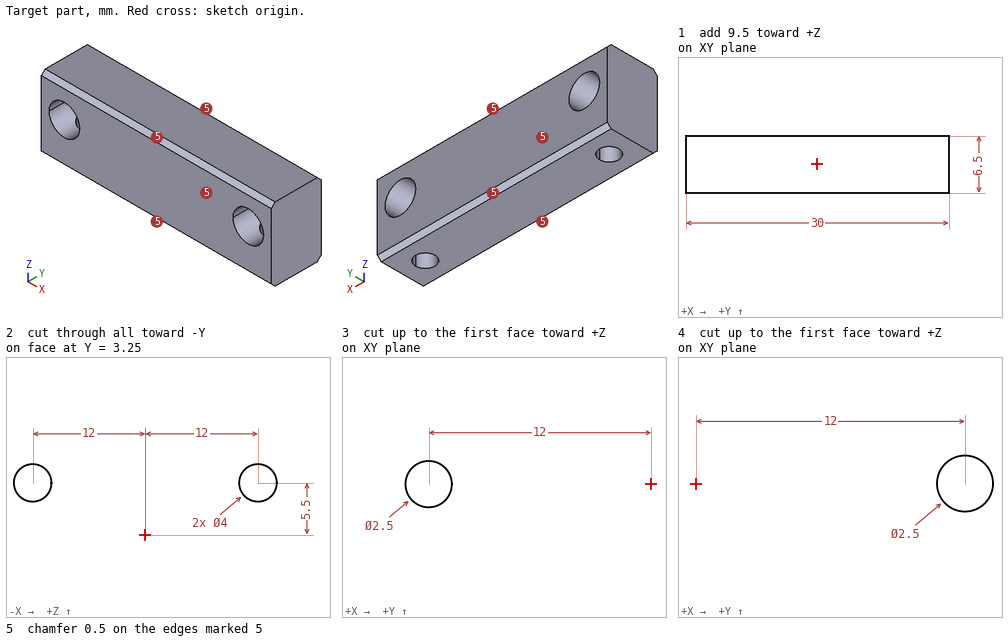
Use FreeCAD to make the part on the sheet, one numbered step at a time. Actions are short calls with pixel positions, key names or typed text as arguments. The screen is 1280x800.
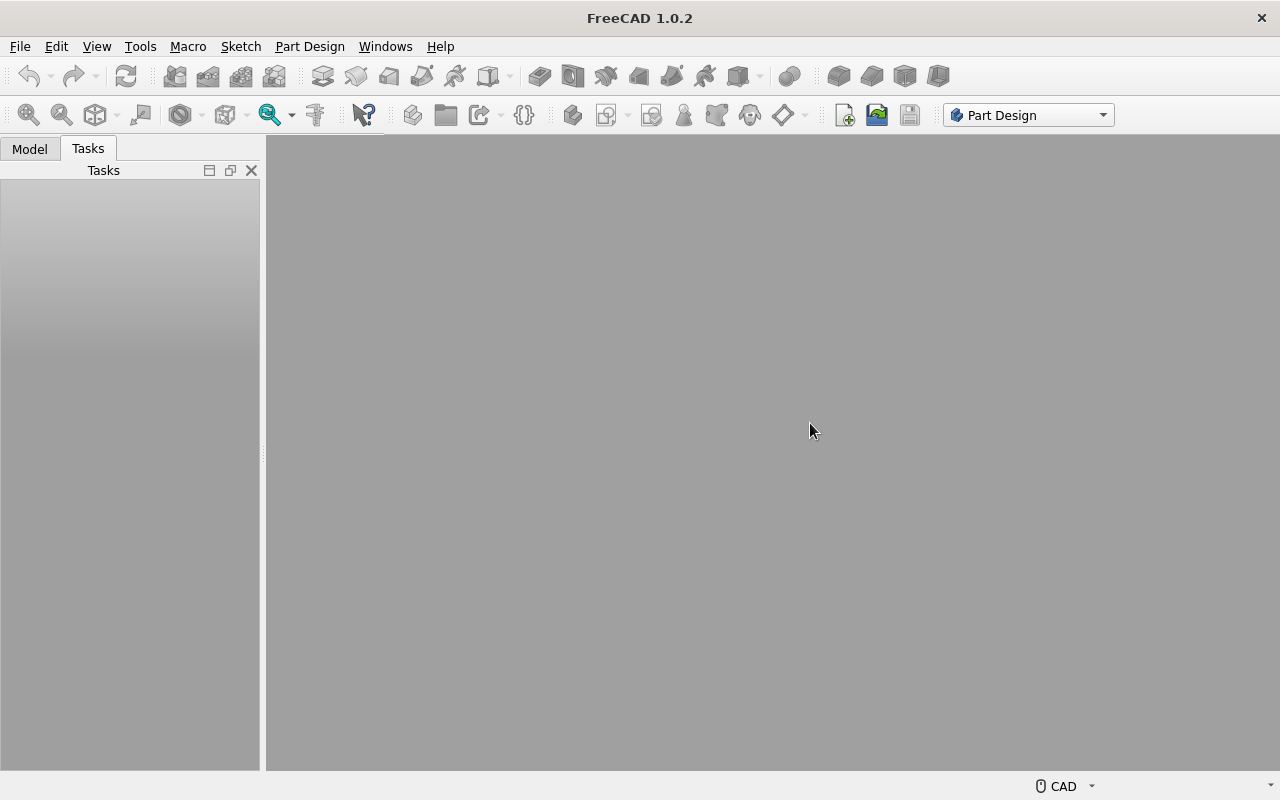
click(844, 116)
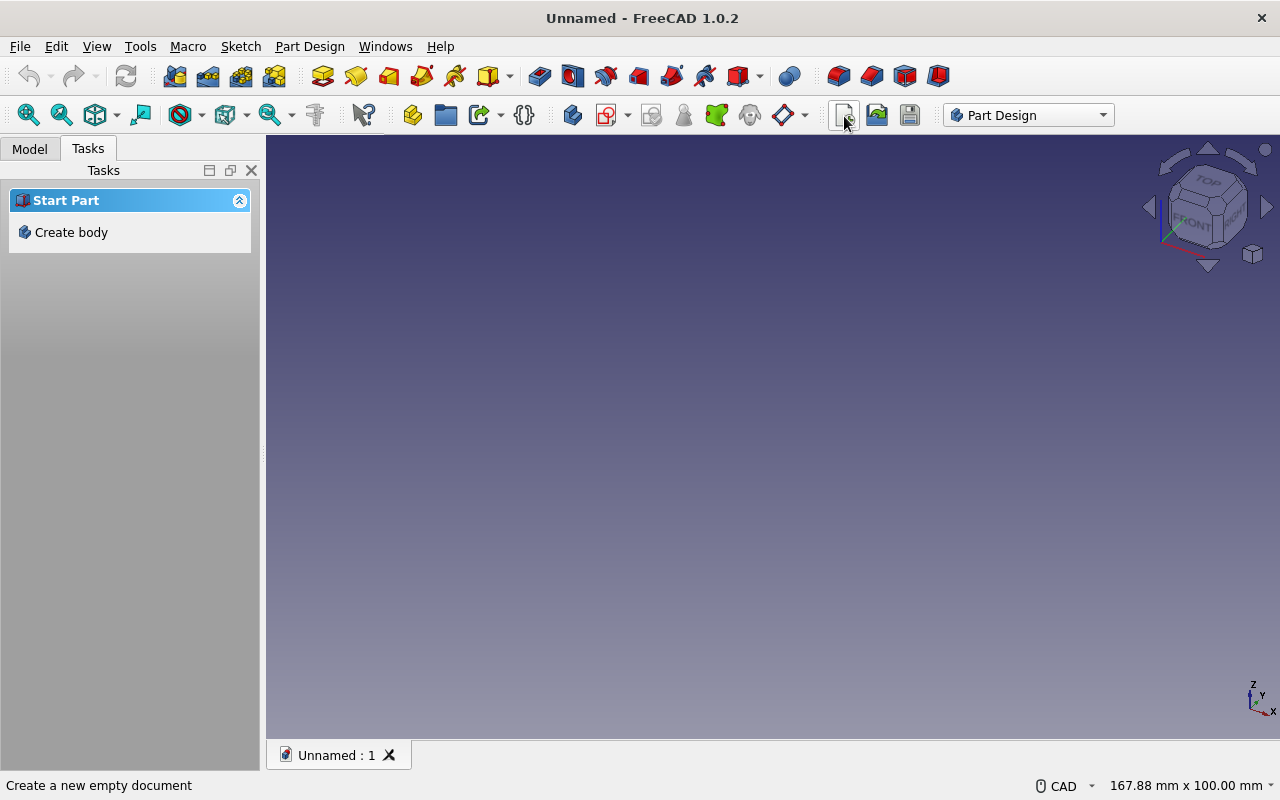
click(606, 116)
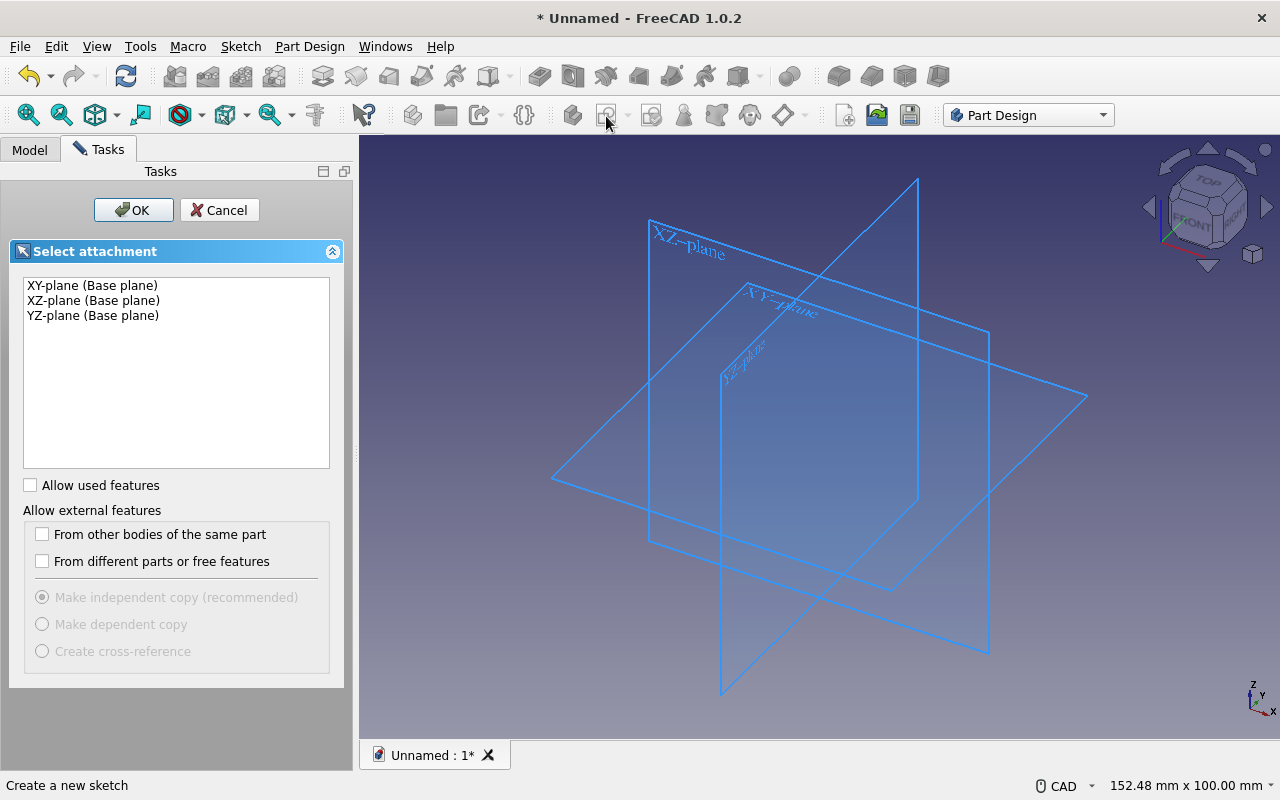
click(84, 286)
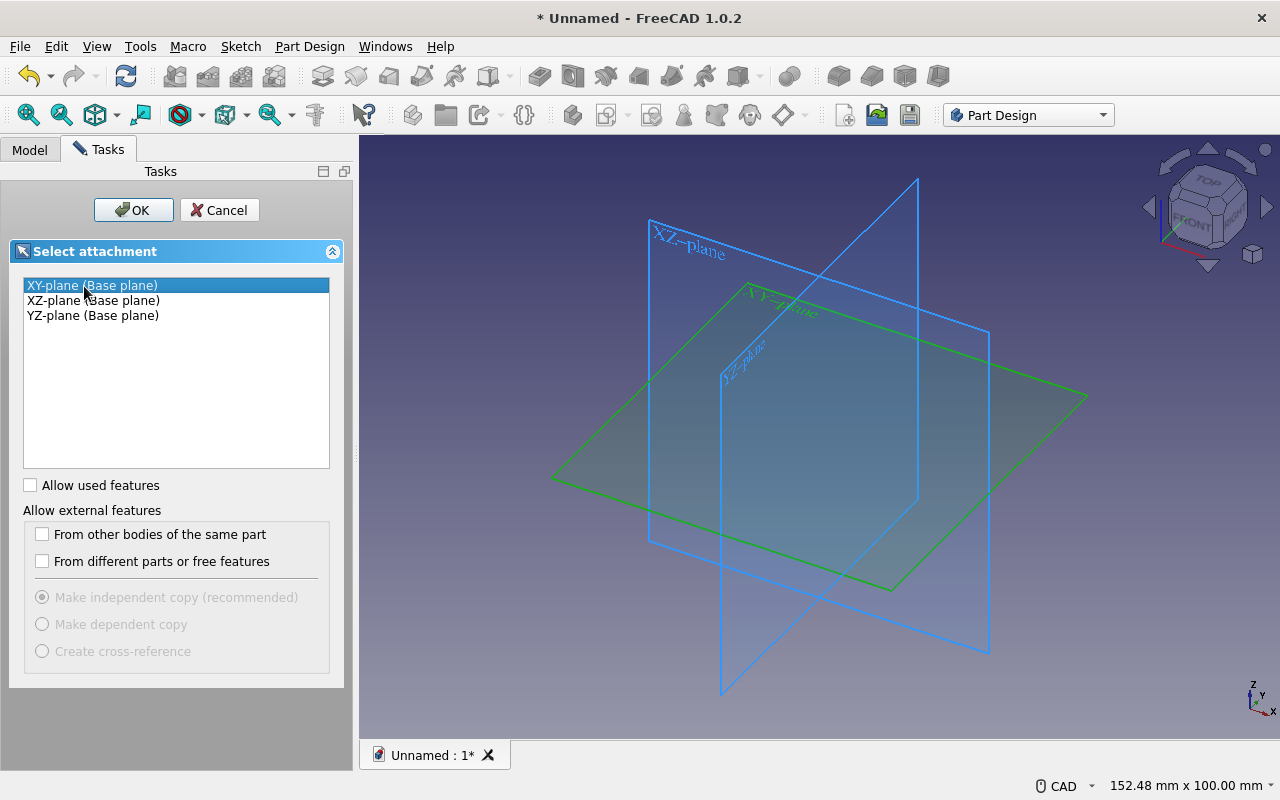
click(134, 210)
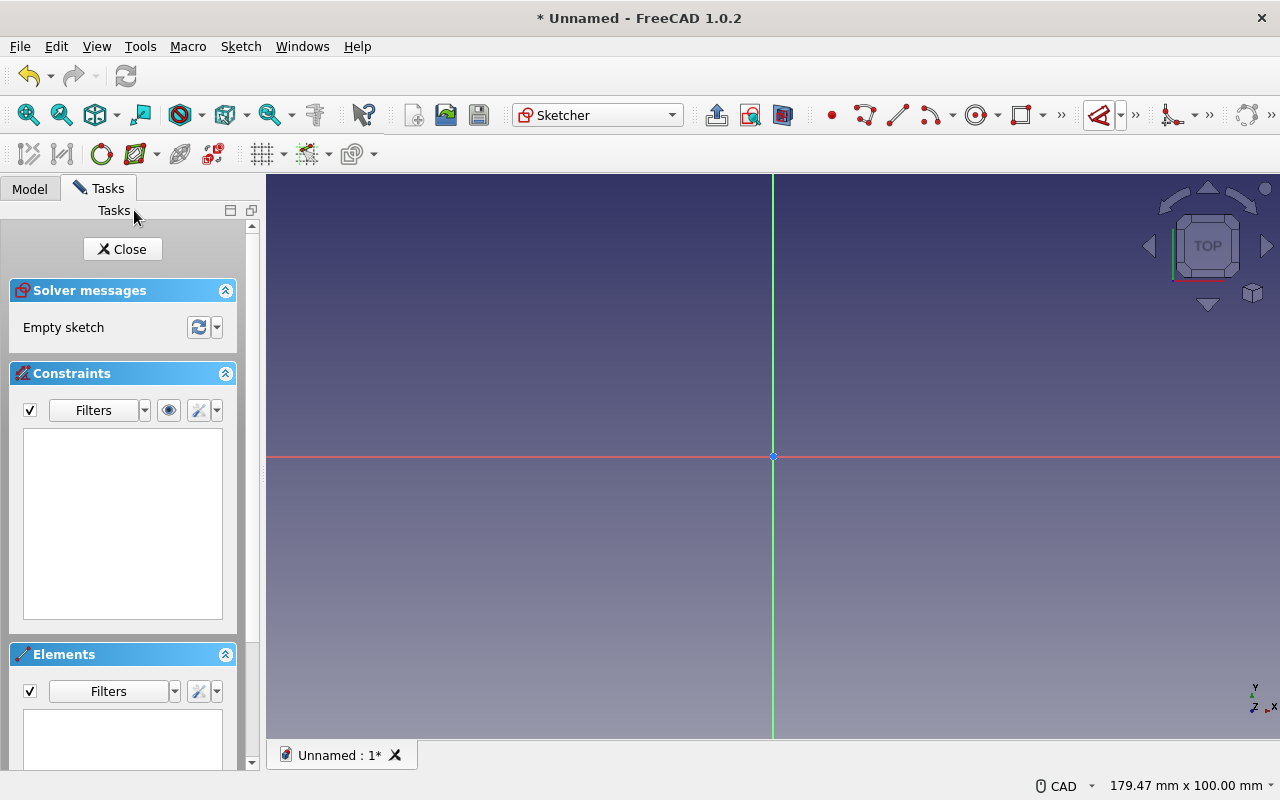
scroll(803, 456, up, 6)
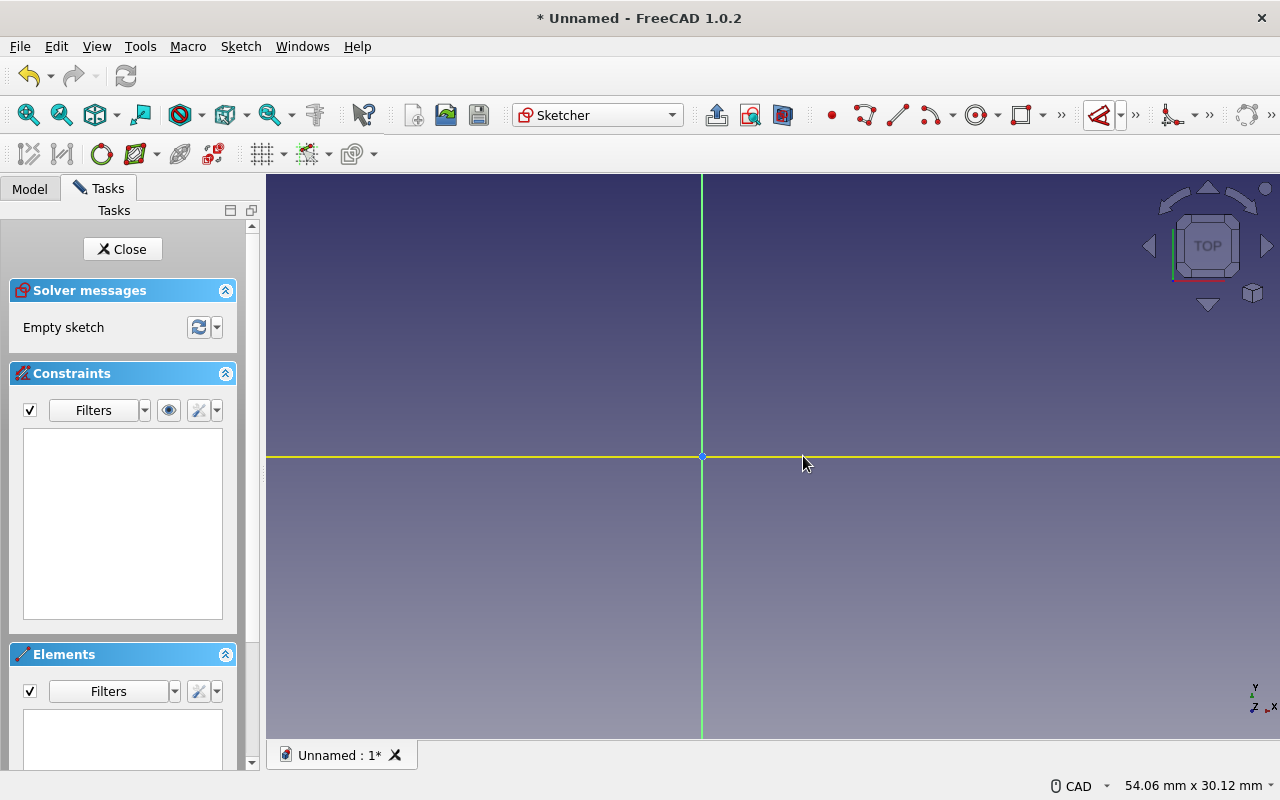
key(g)
key(v)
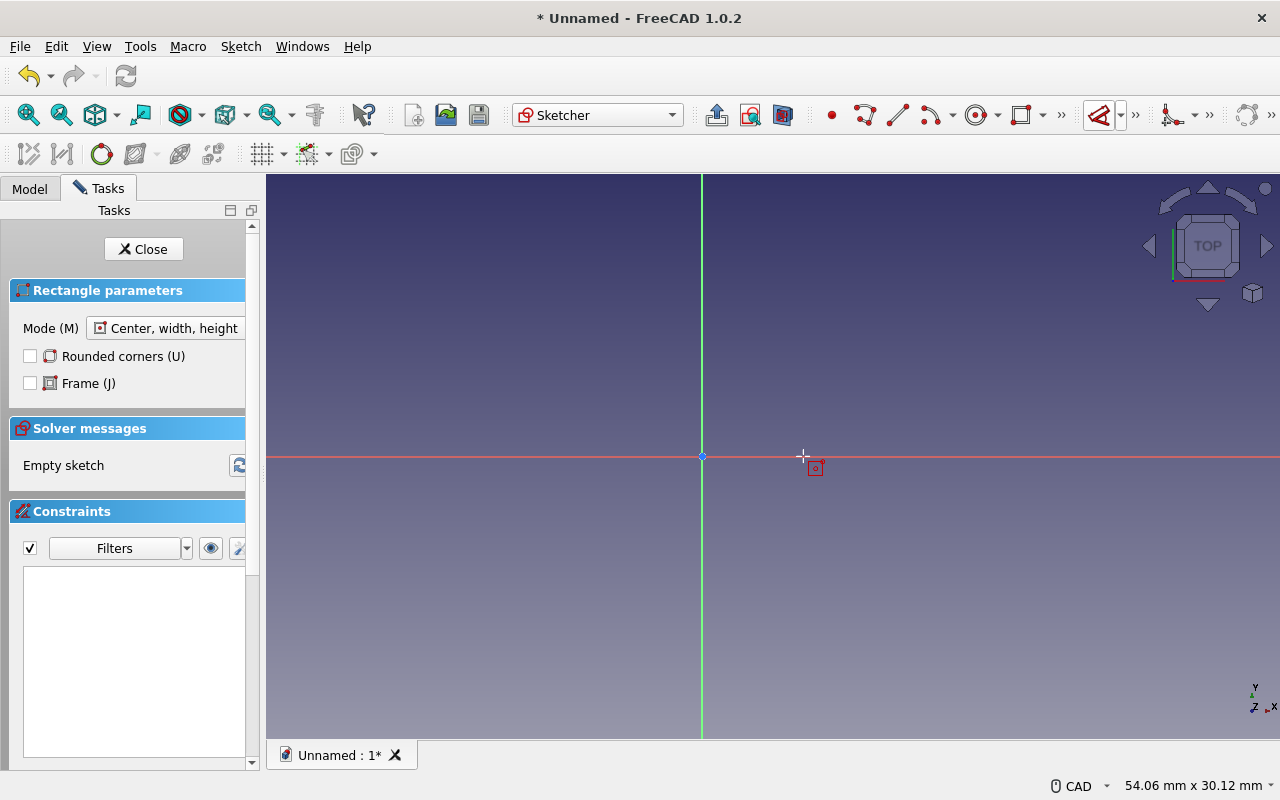
click(702, 456)
click(984, 396)
key(Escape)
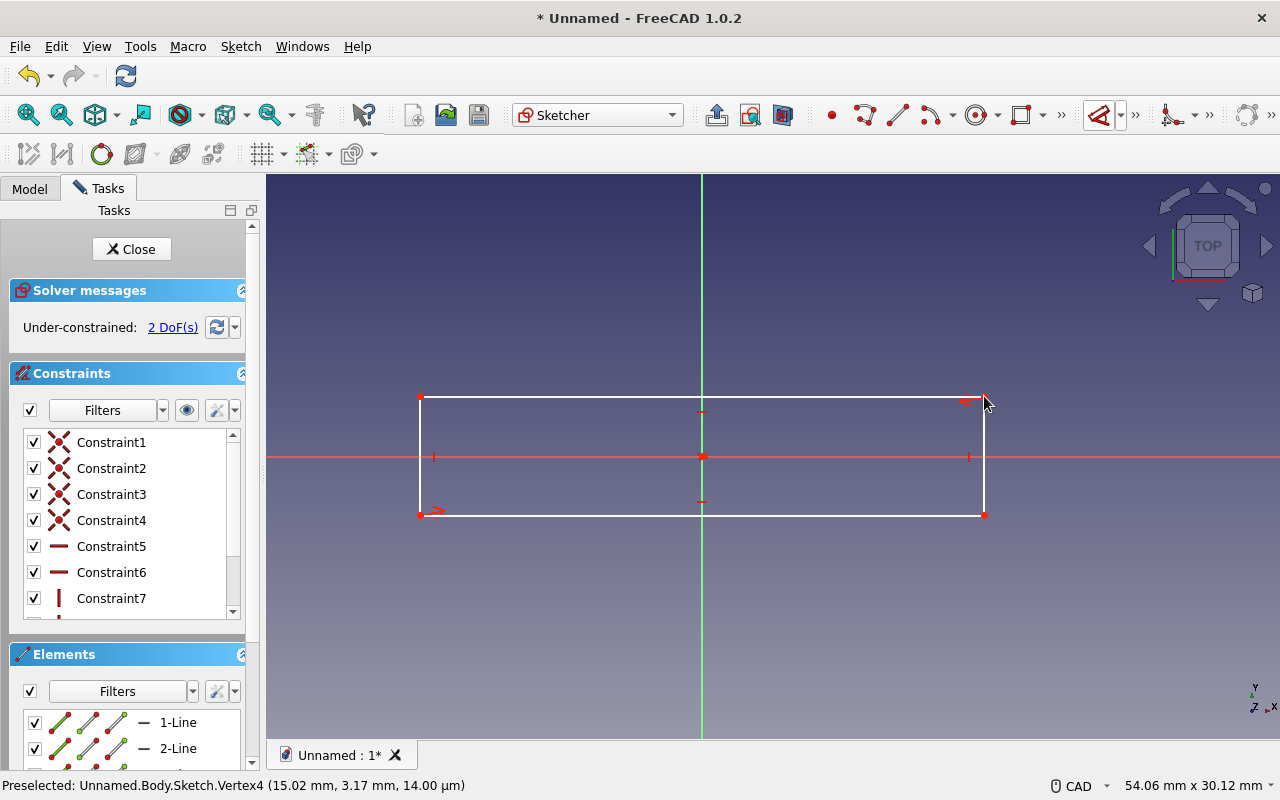
click(1098, 116)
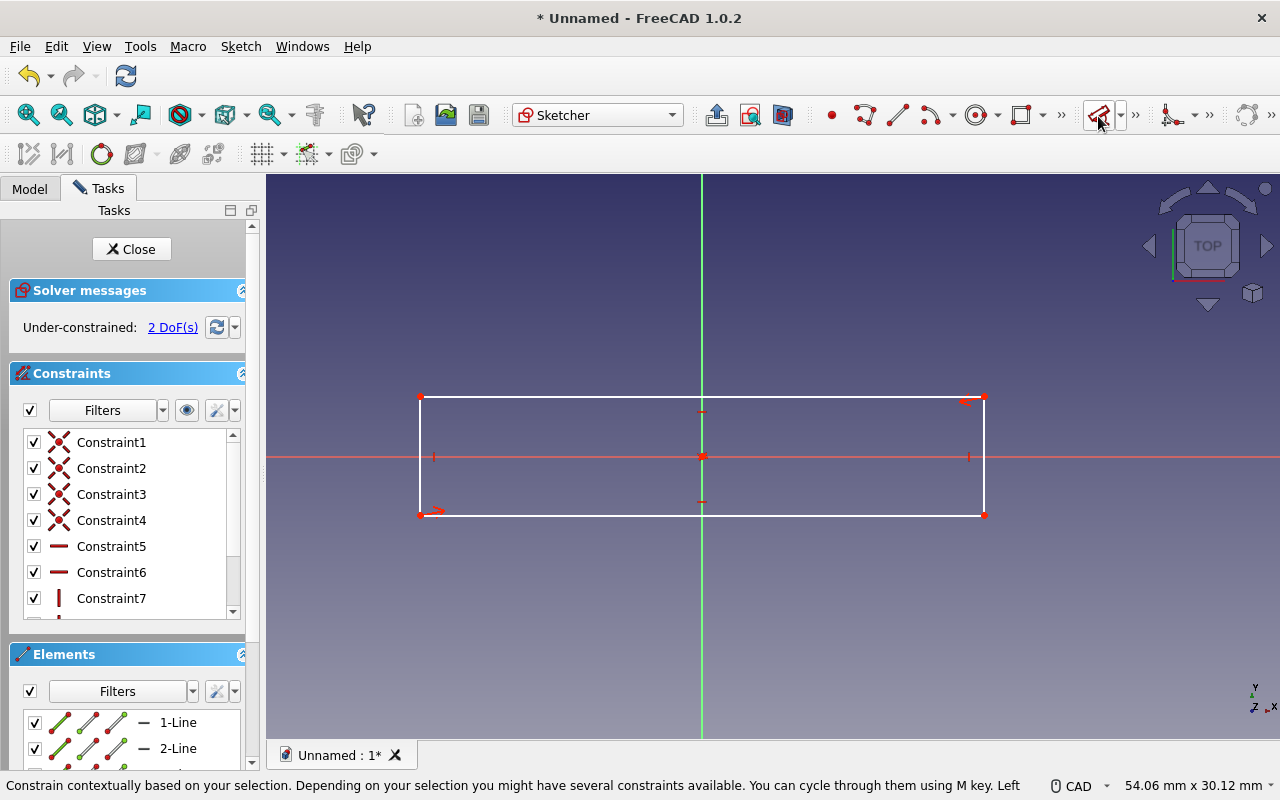
click(589, 516)
click(573, 550)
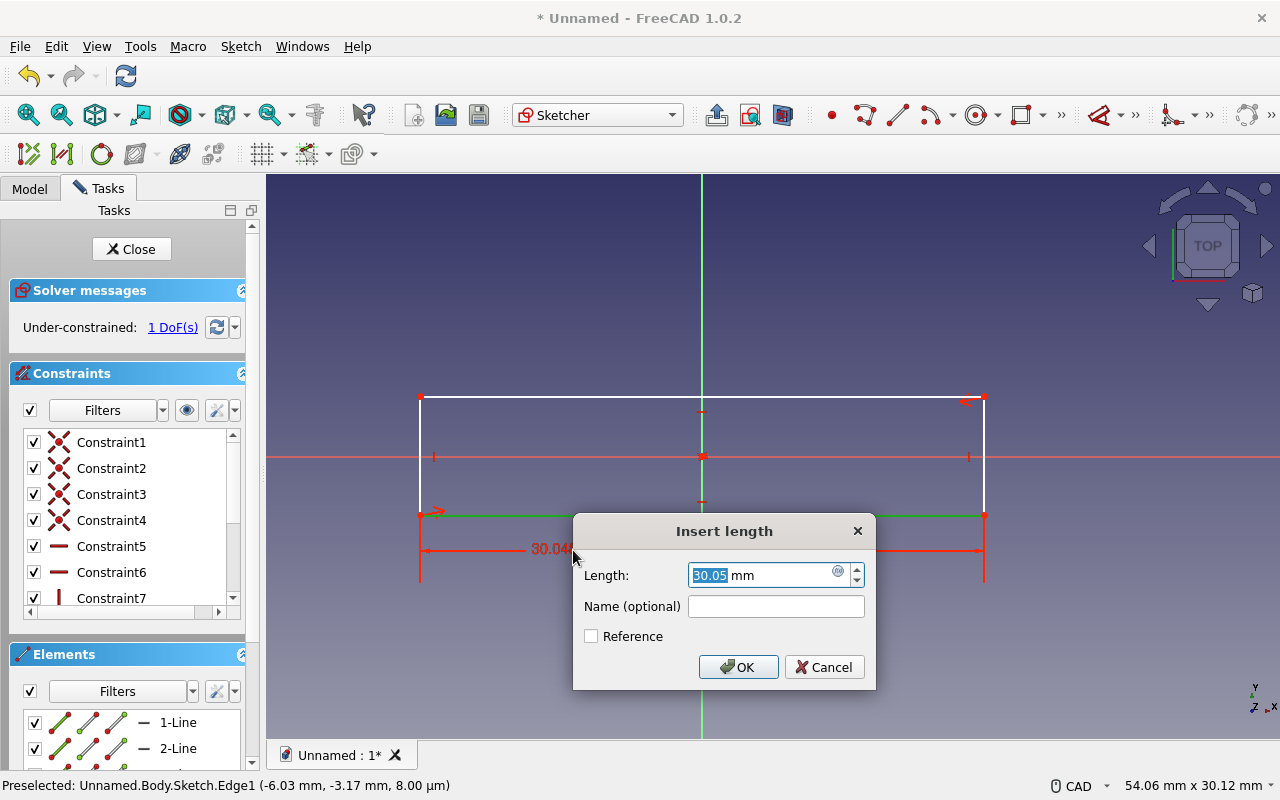
text(30)
key(Return)